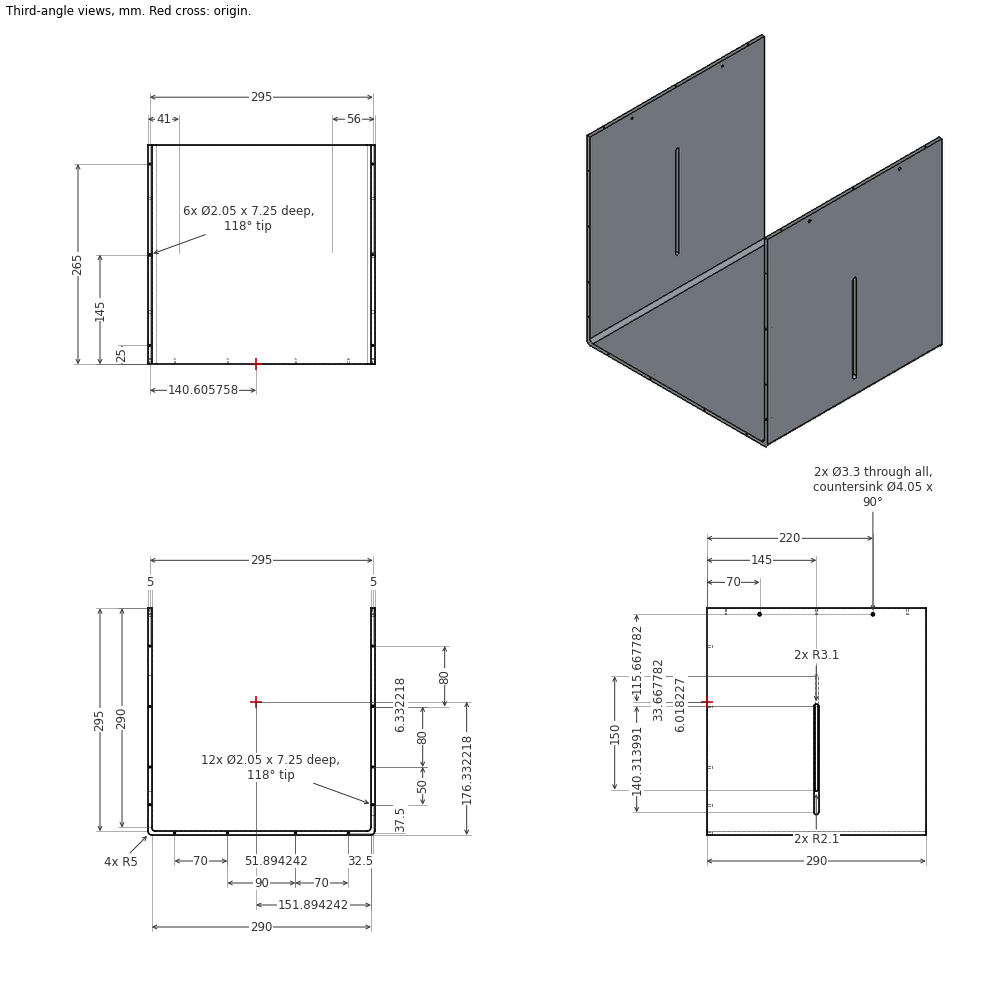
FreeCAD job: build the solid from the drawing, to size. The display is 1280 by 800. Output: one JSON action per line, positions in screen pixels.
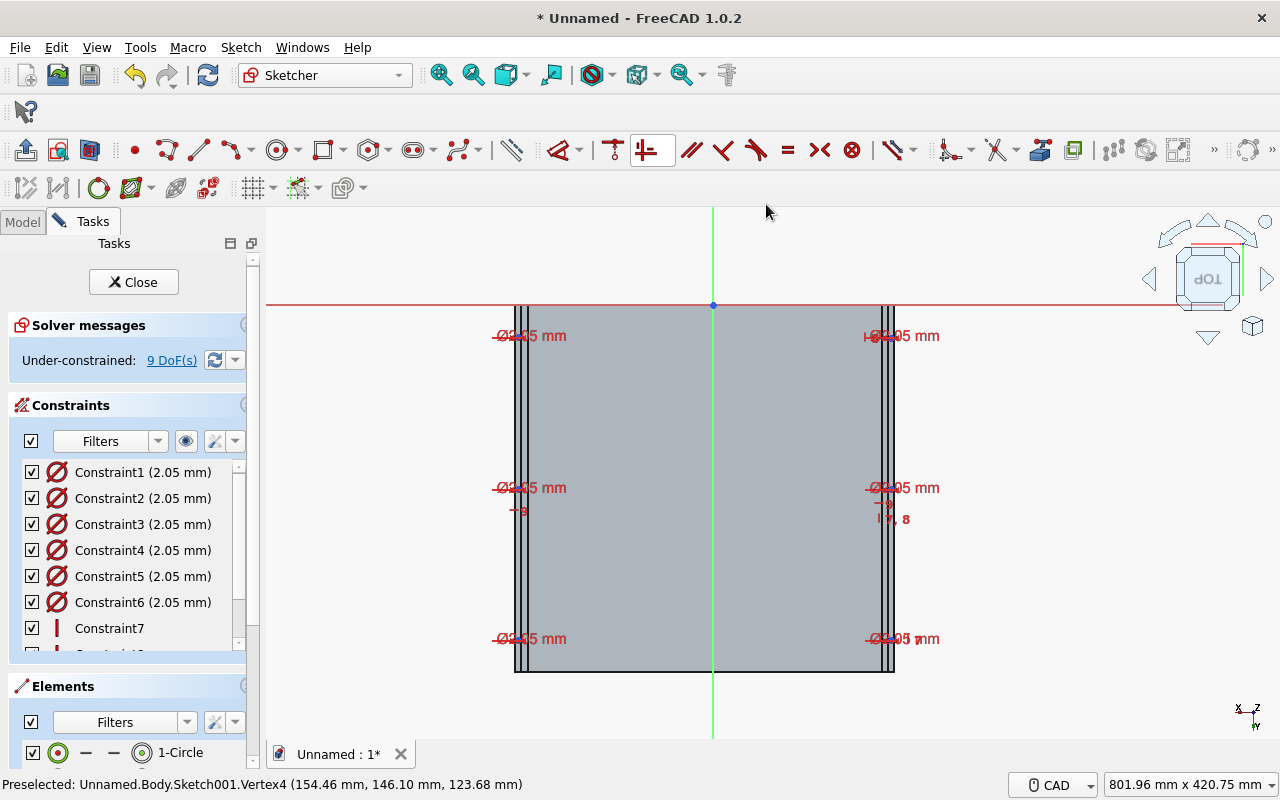
{"action": "left_click", "coordinate": [518, 490]}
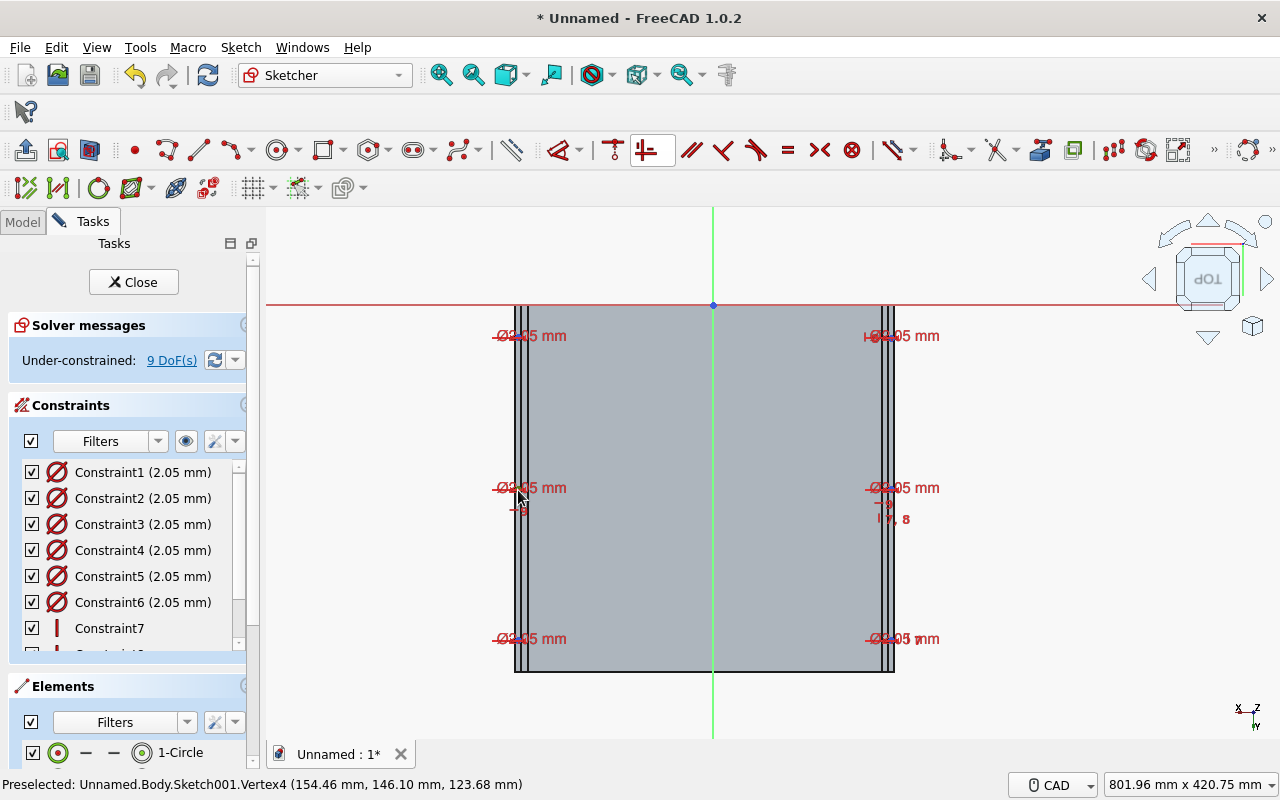
{"action": "left_click", "coordinate": [518, 641]}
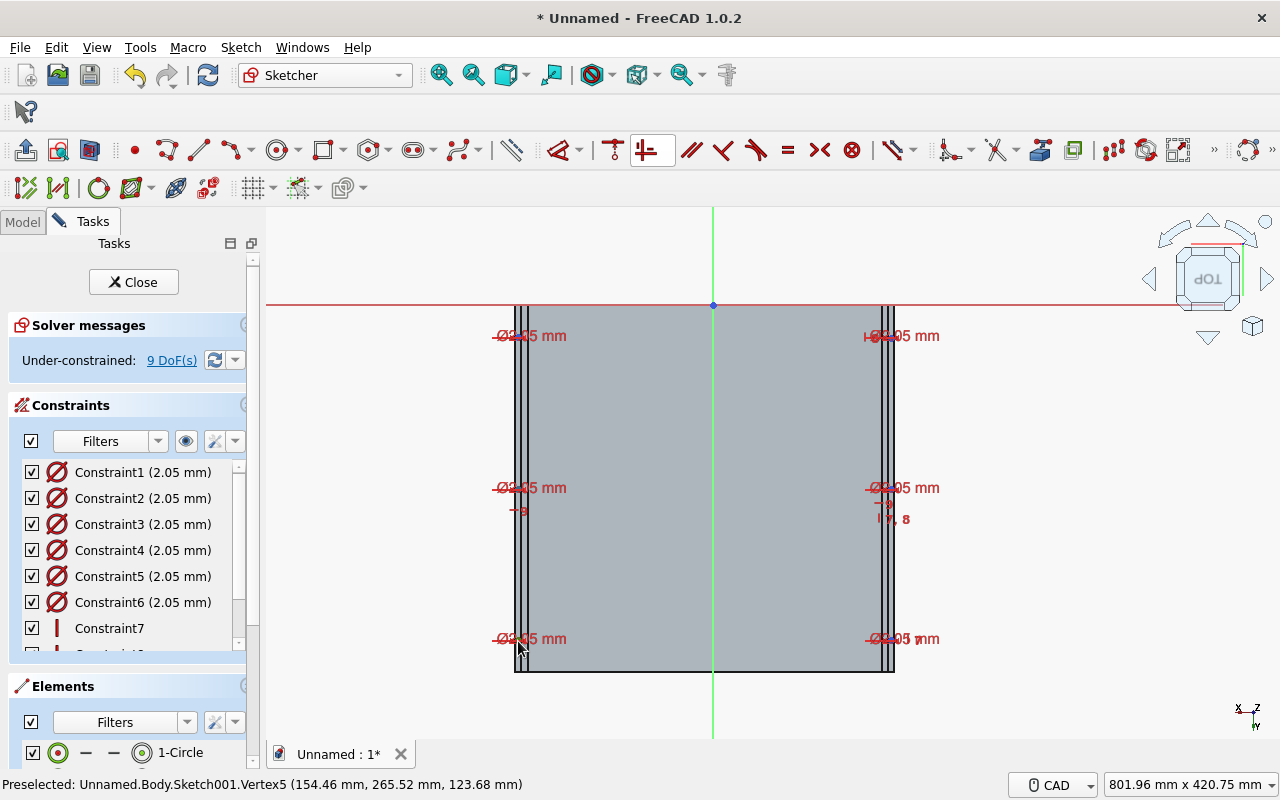
{"action": "key", "text": "v"}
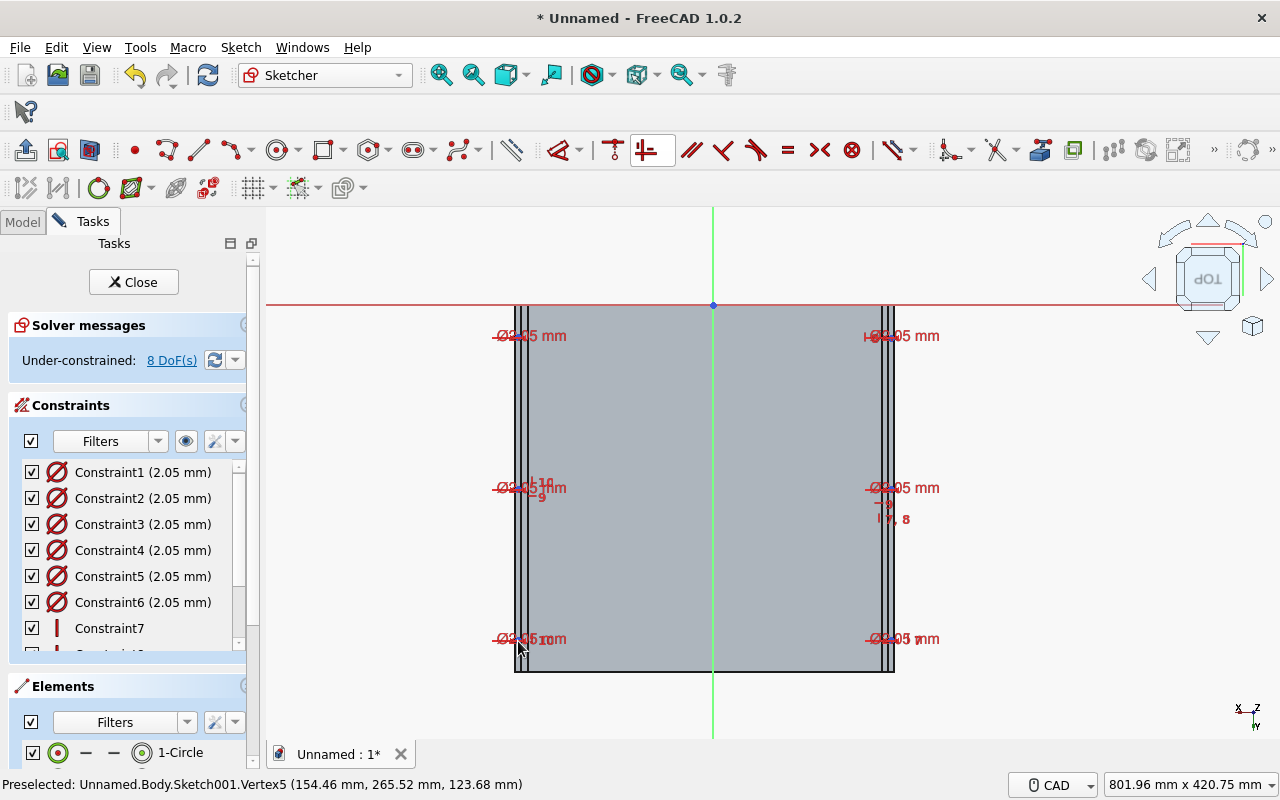
{"action": "left_click", "coordinate": [891, 641]}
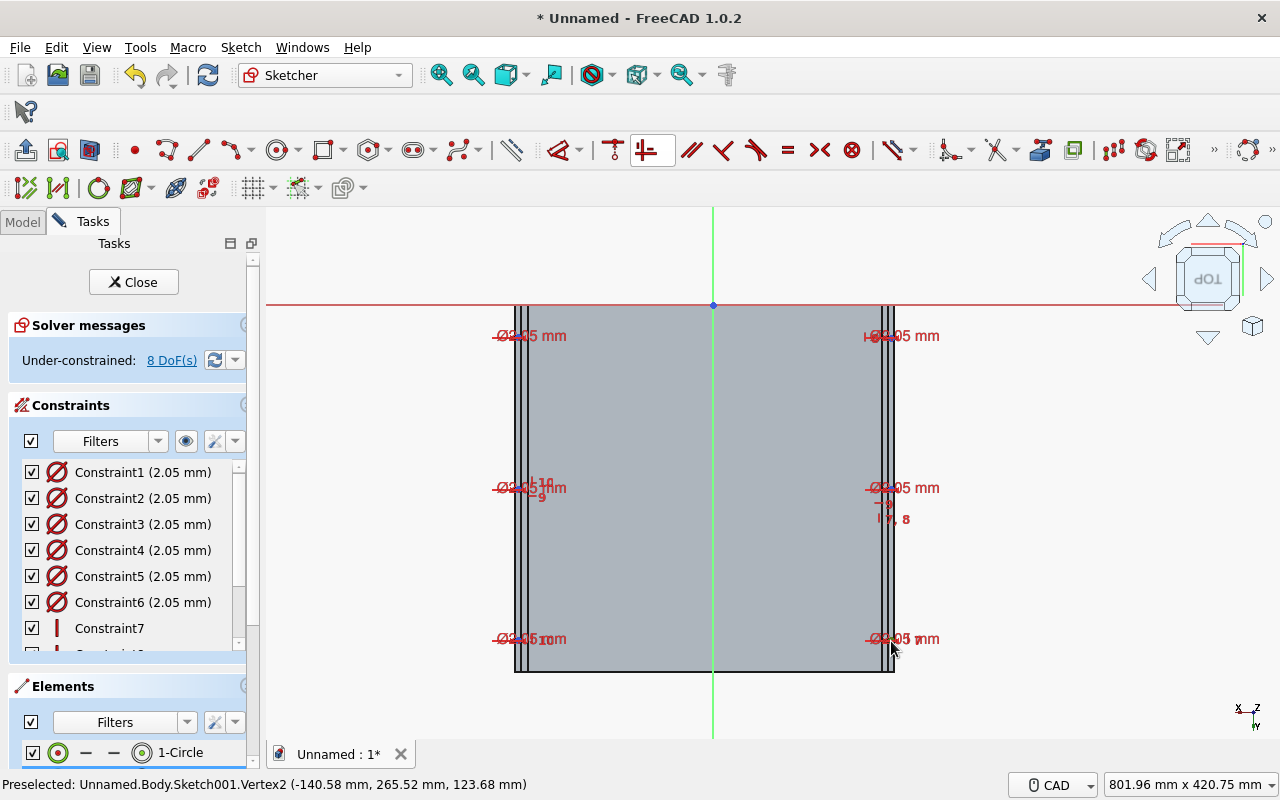
{"action": "left_click", "coordinate": [518, 641]}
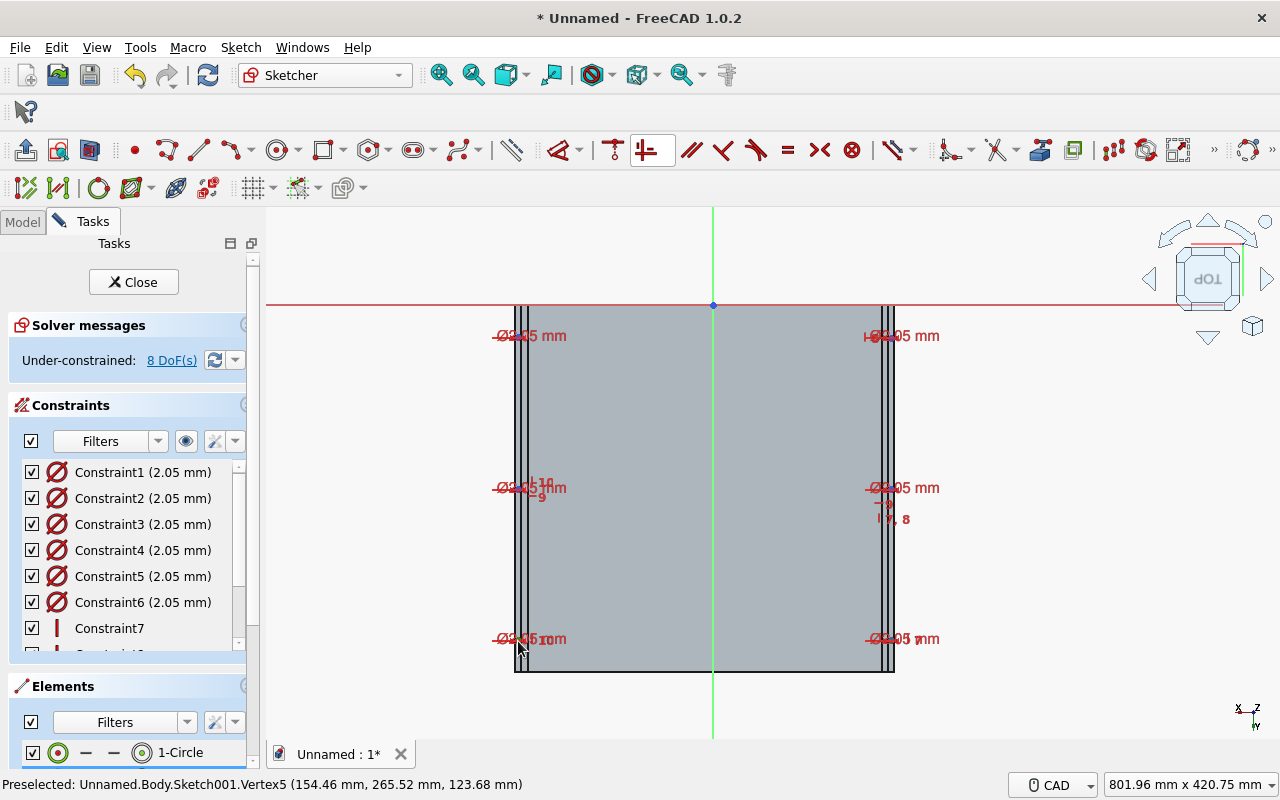
{"action": "left_click", "coordinate": [670, 150]}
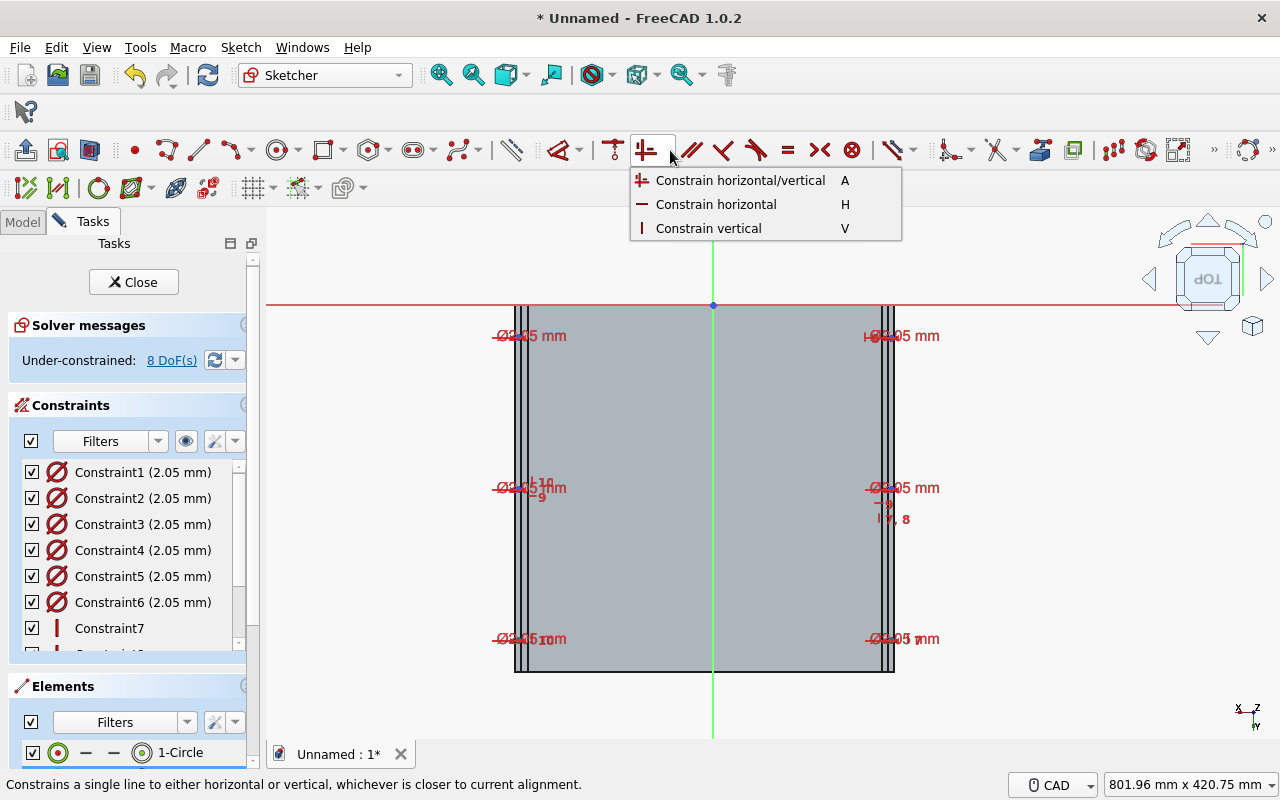
{"action": "left_click", "coordinate": [766, 204]}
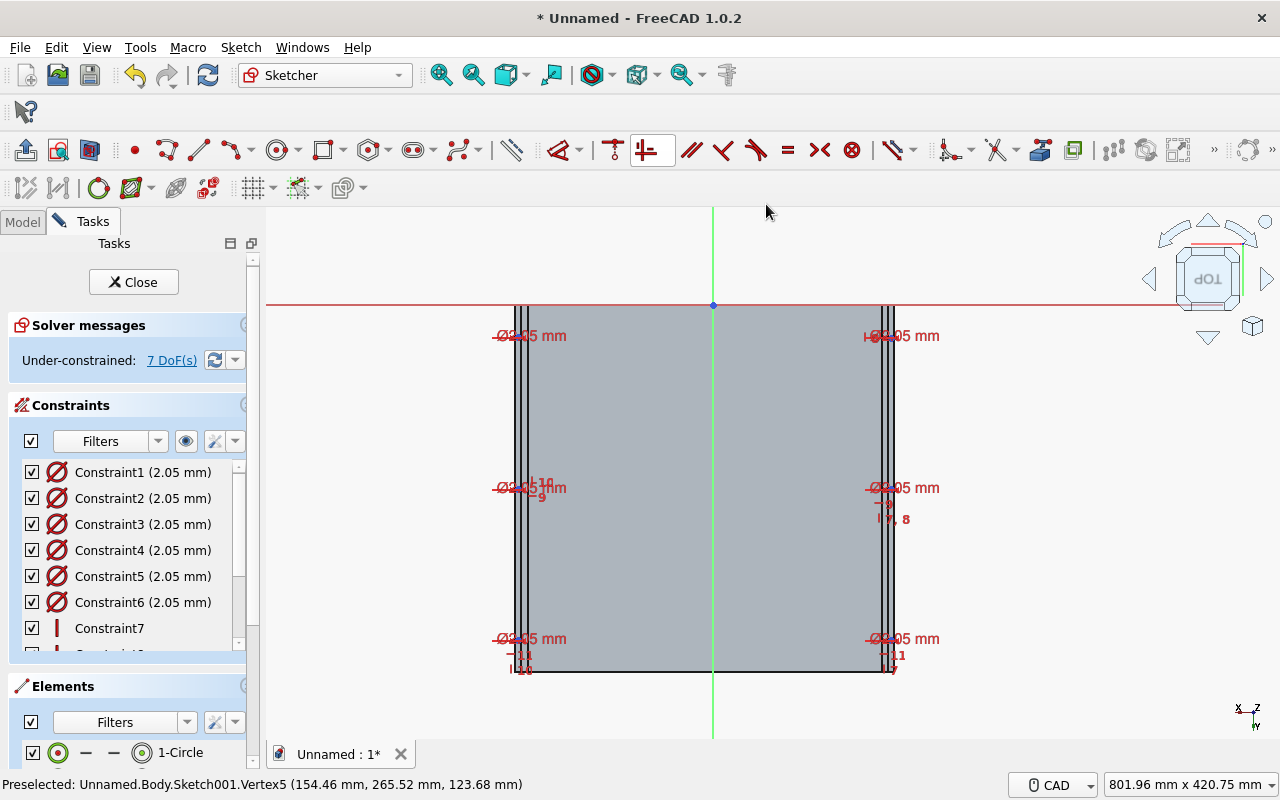
{"action": "left_click", "coordinate": [518, 490]}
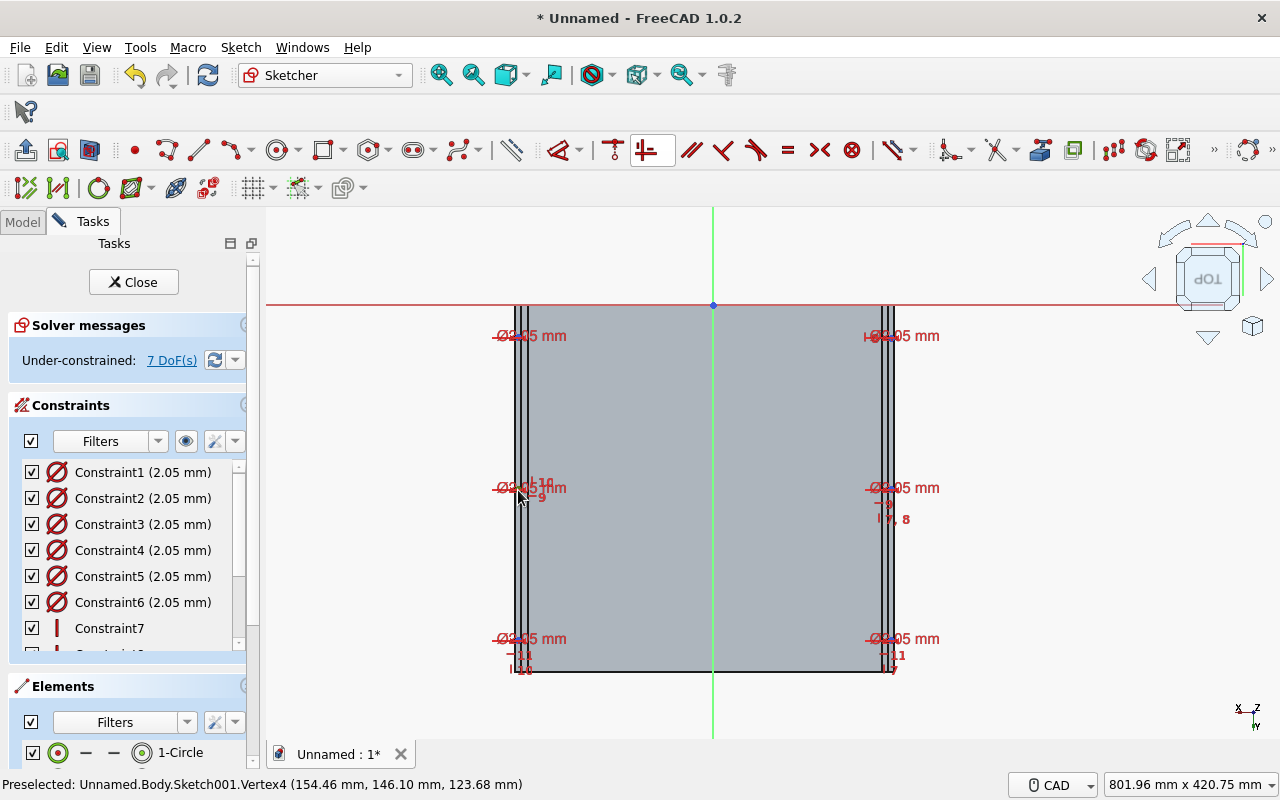
{"action": "left_click", "coordinate": [518, 338]}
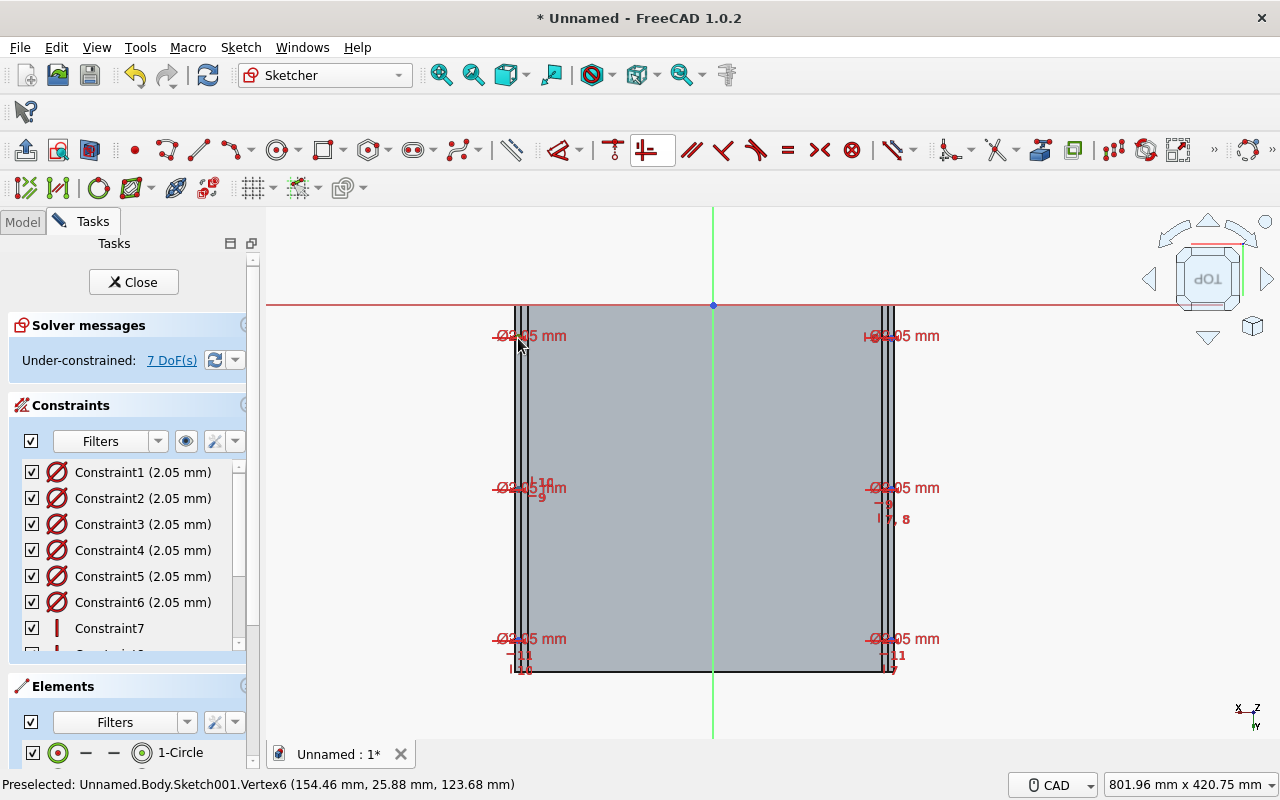
{"action": "left_click", "coordinate": [670, 150]}